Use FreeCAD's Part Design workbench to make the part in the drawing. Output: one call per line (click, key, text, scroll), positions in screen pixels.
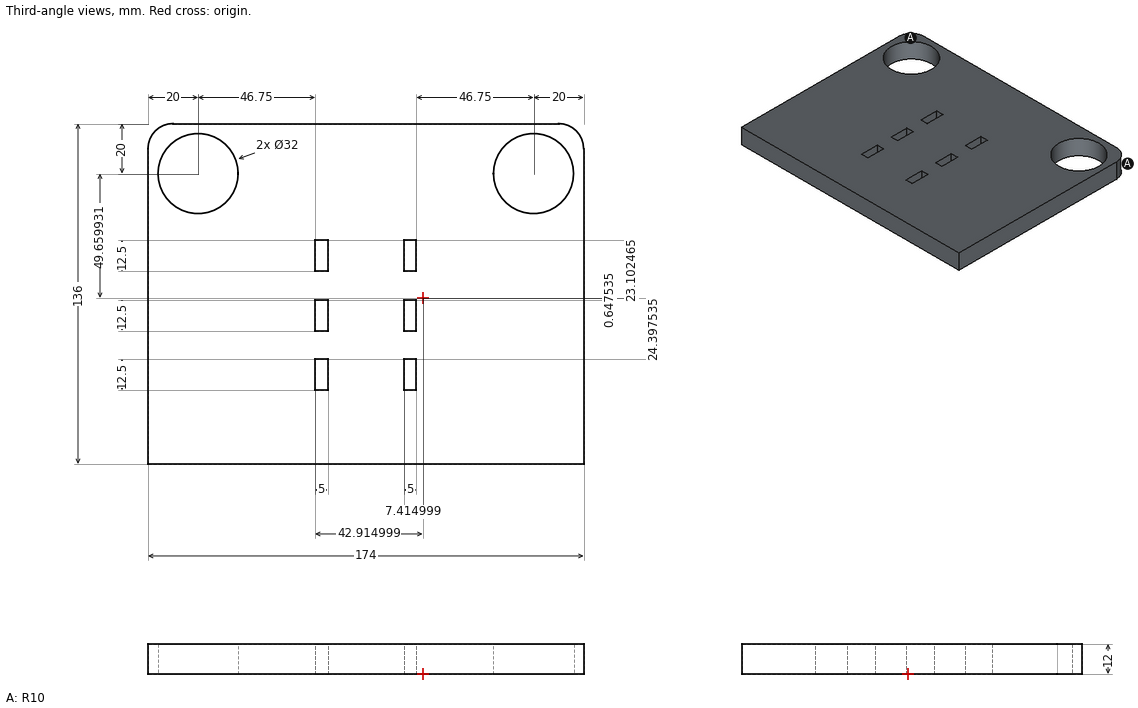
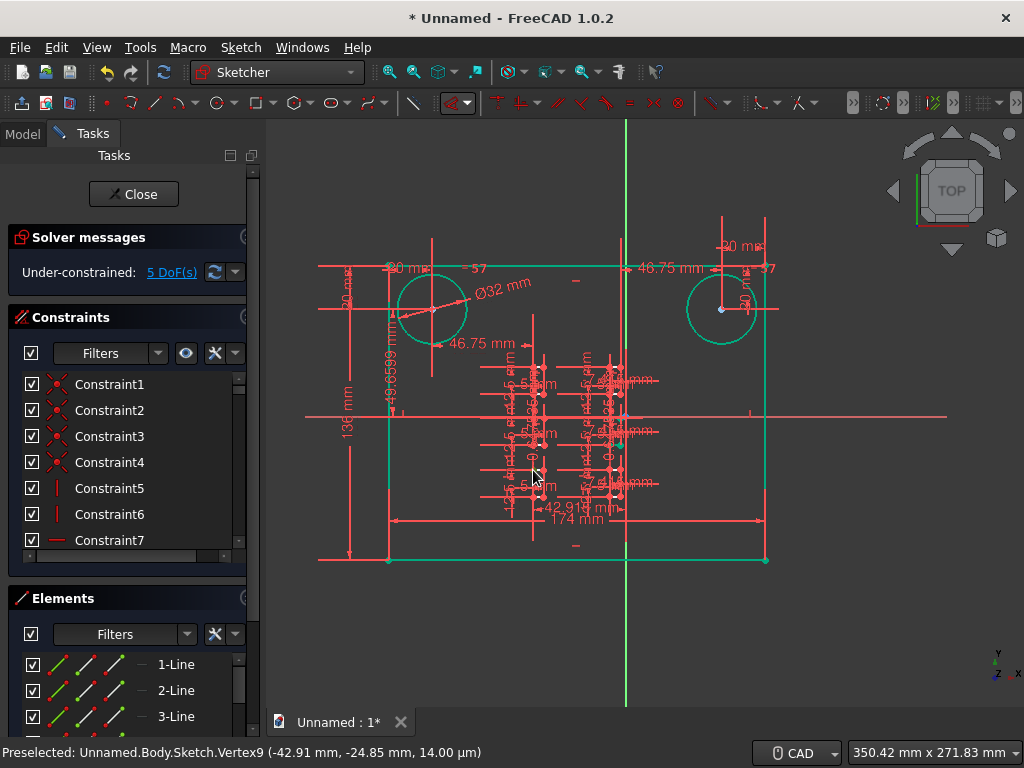
click(470, 104)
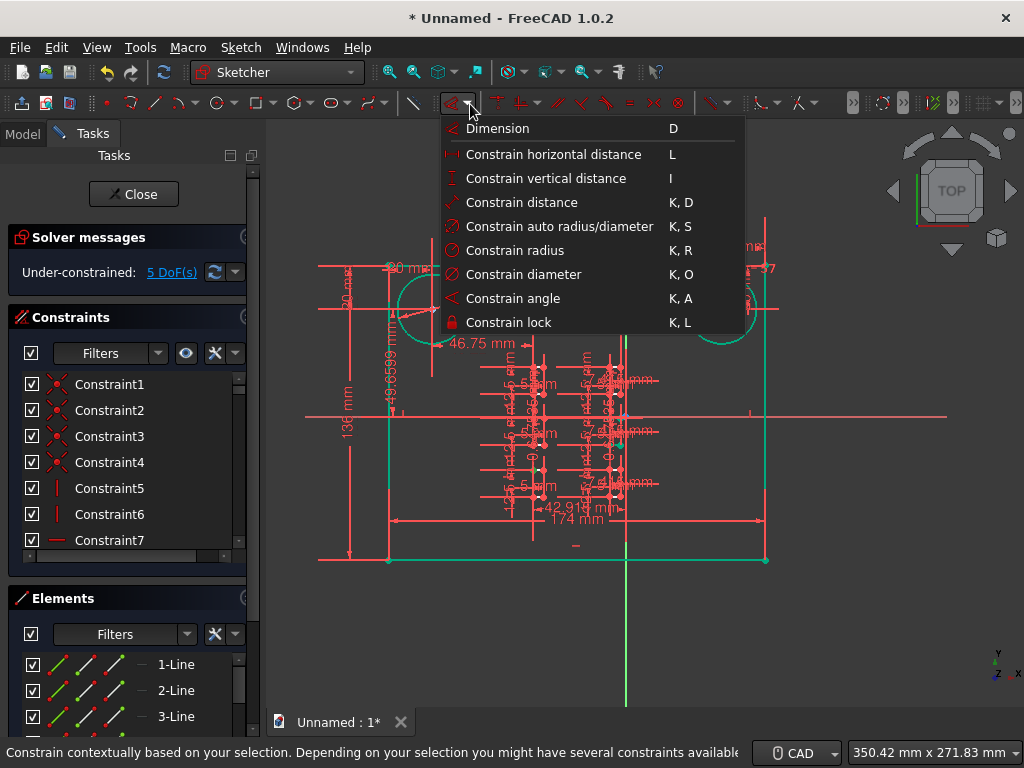
click(593, 178)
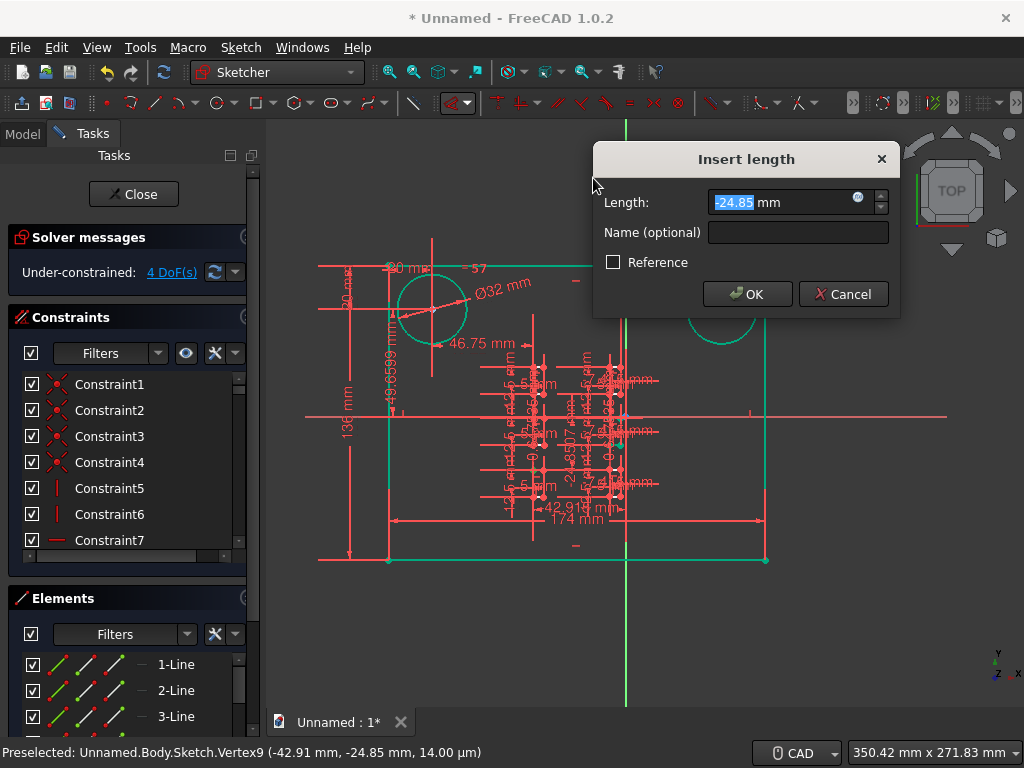
text(-24.397535)
key(Return)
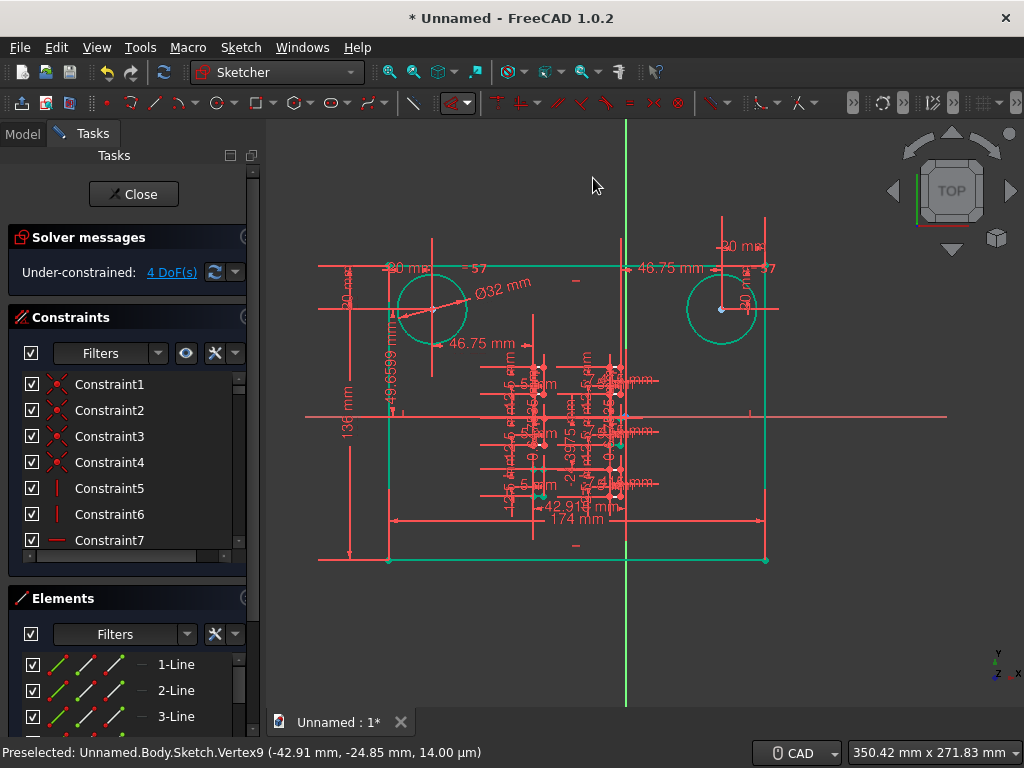
click(533, 418)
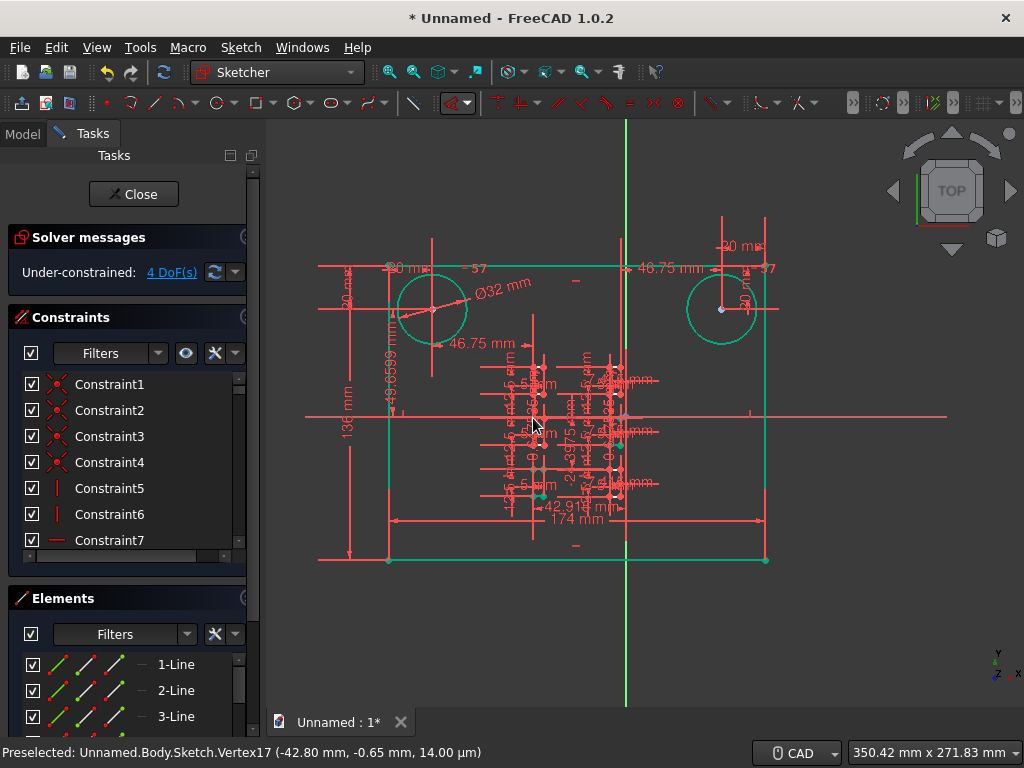
key(l)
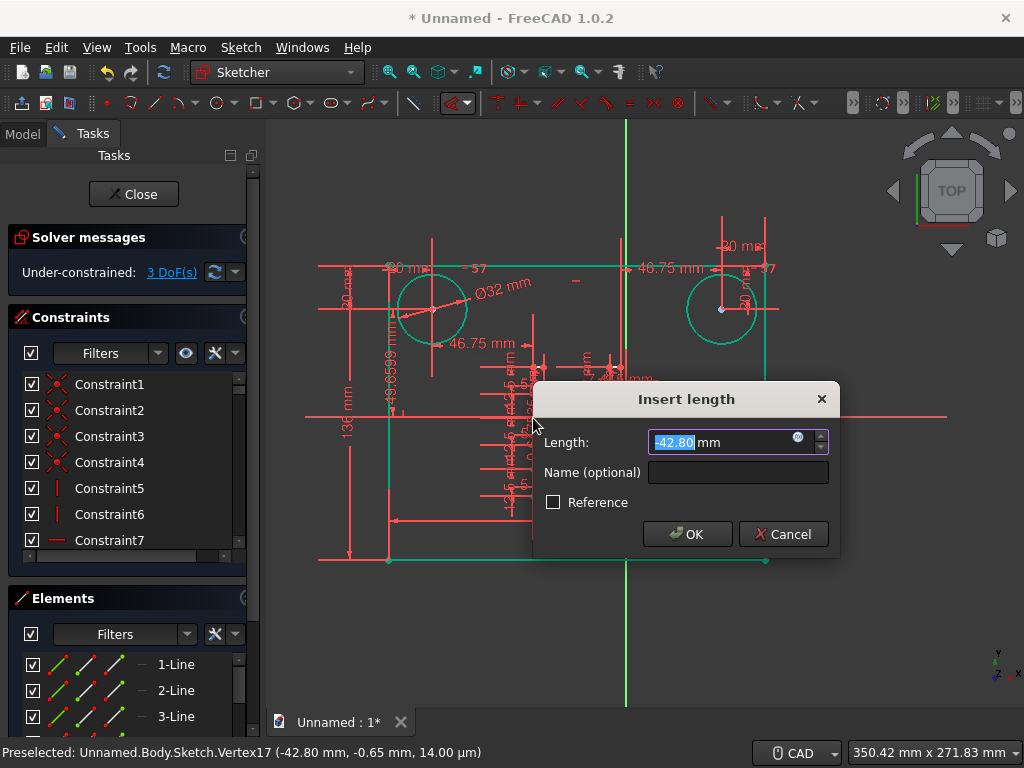
text(-42.914999)
key(Return)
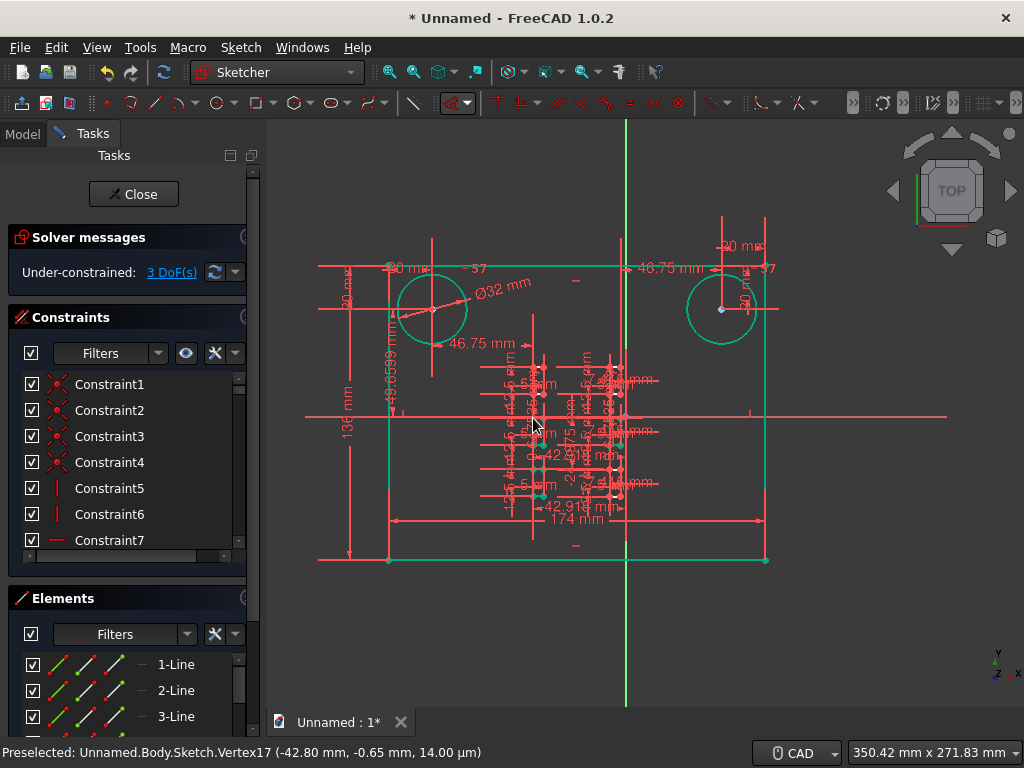
click(610, 470)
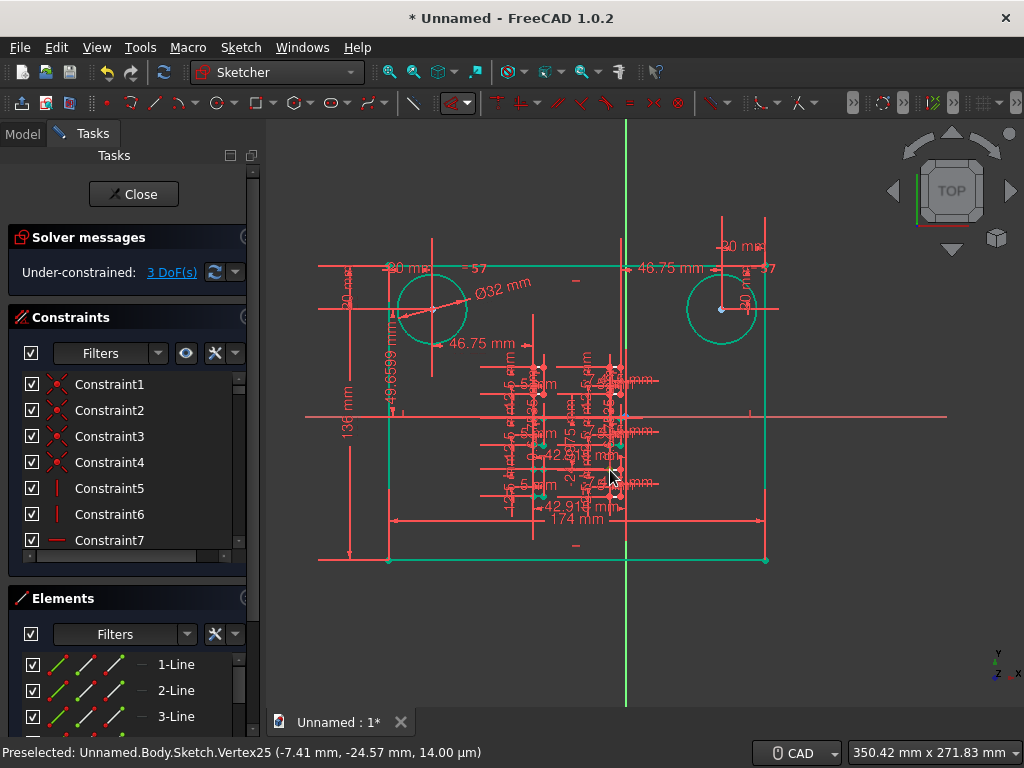
key(i)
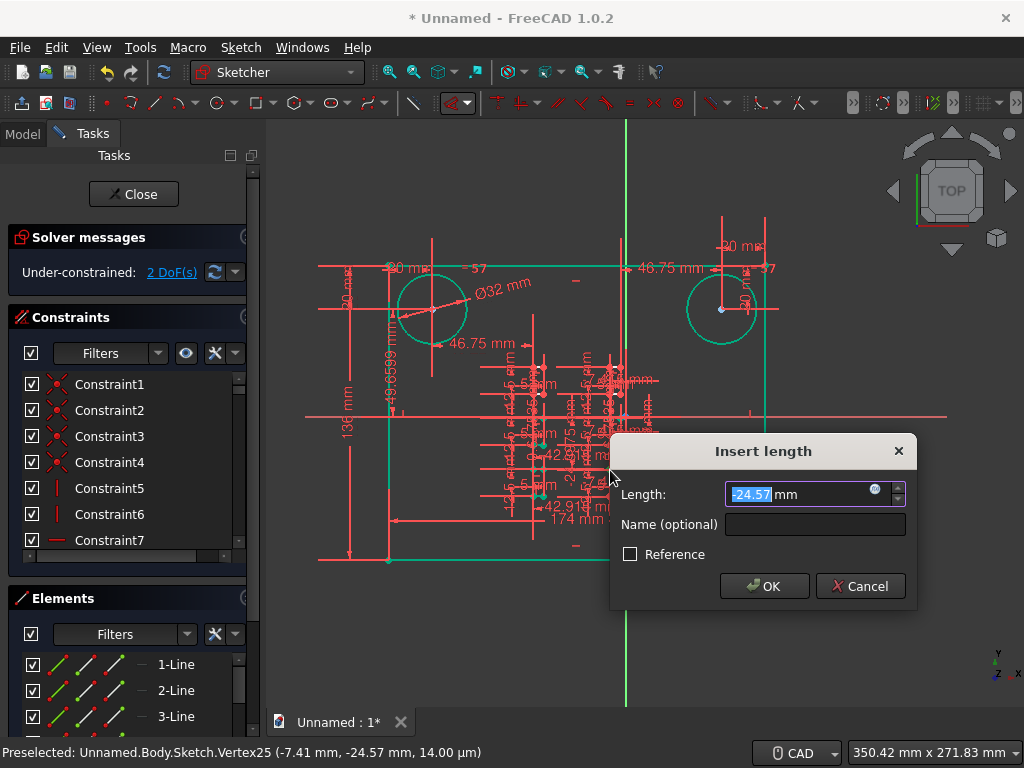
text(-24.397535)
key(Return)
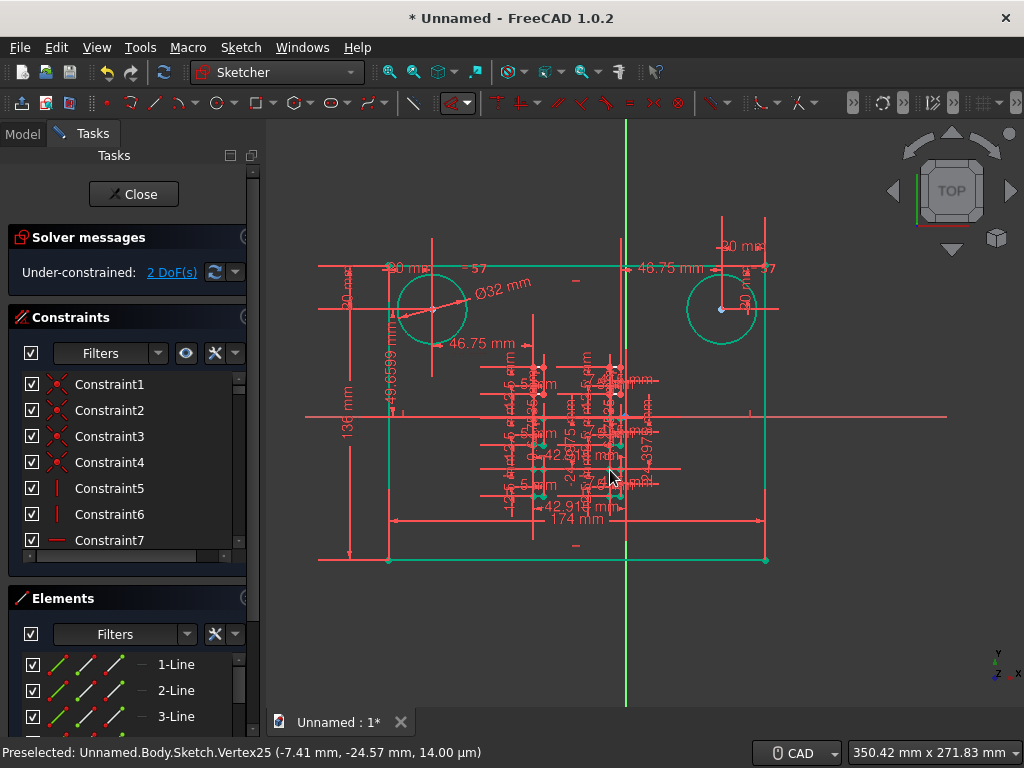
click(533, 367)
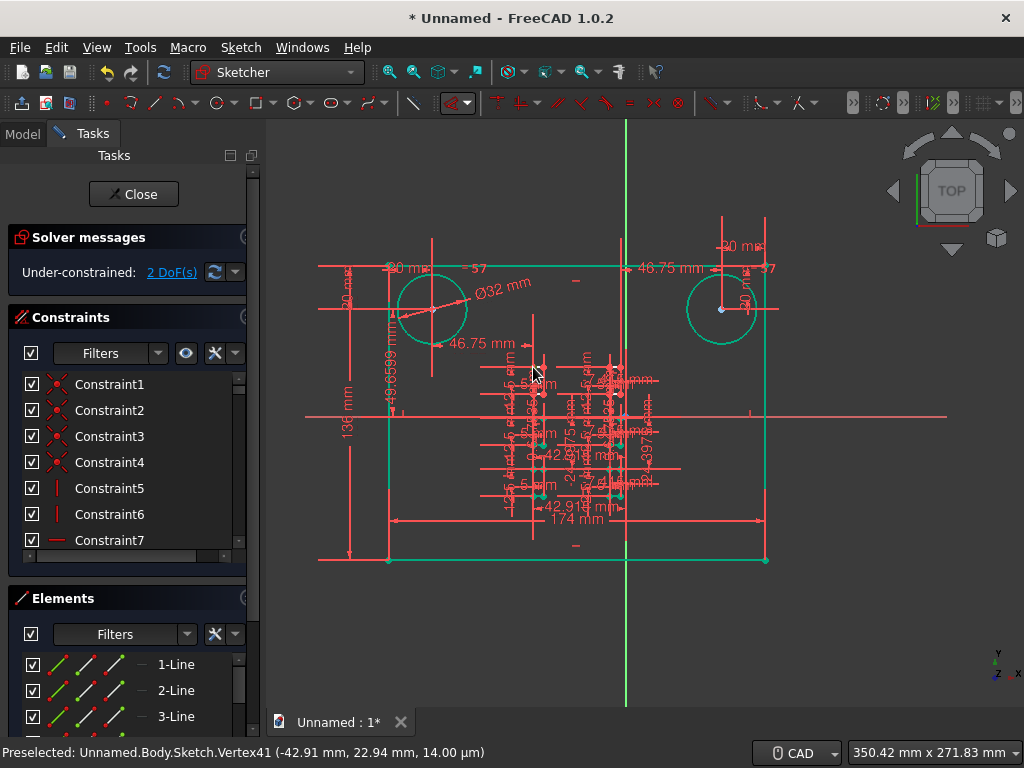
click(470, 104)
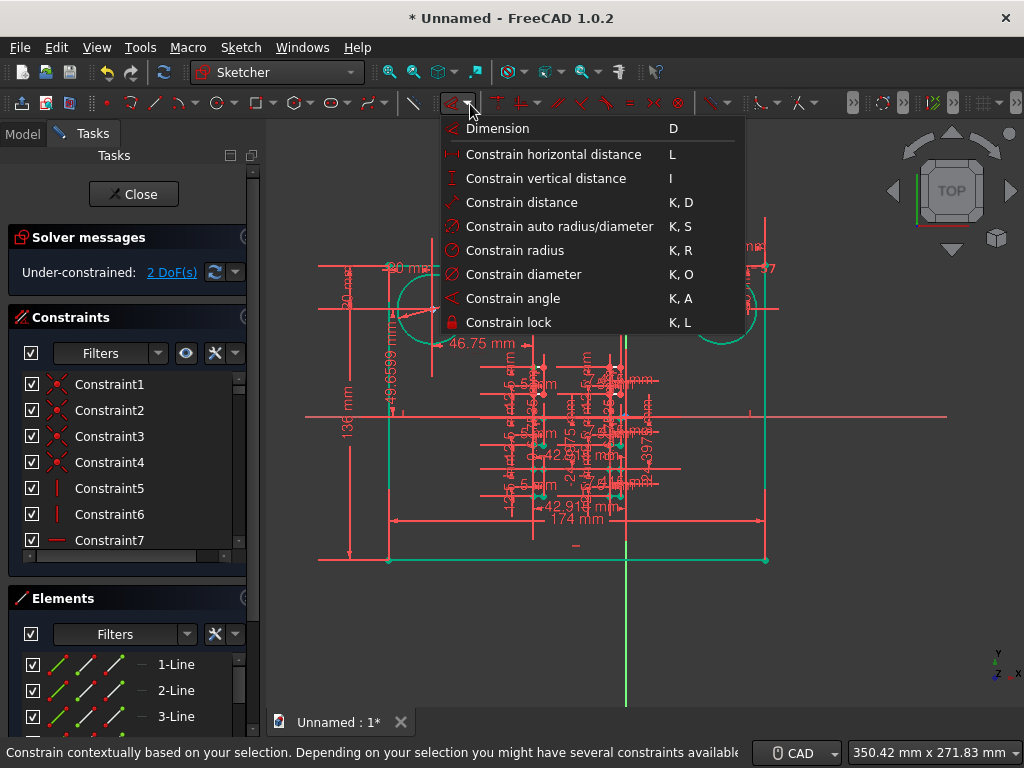
click(593, 178)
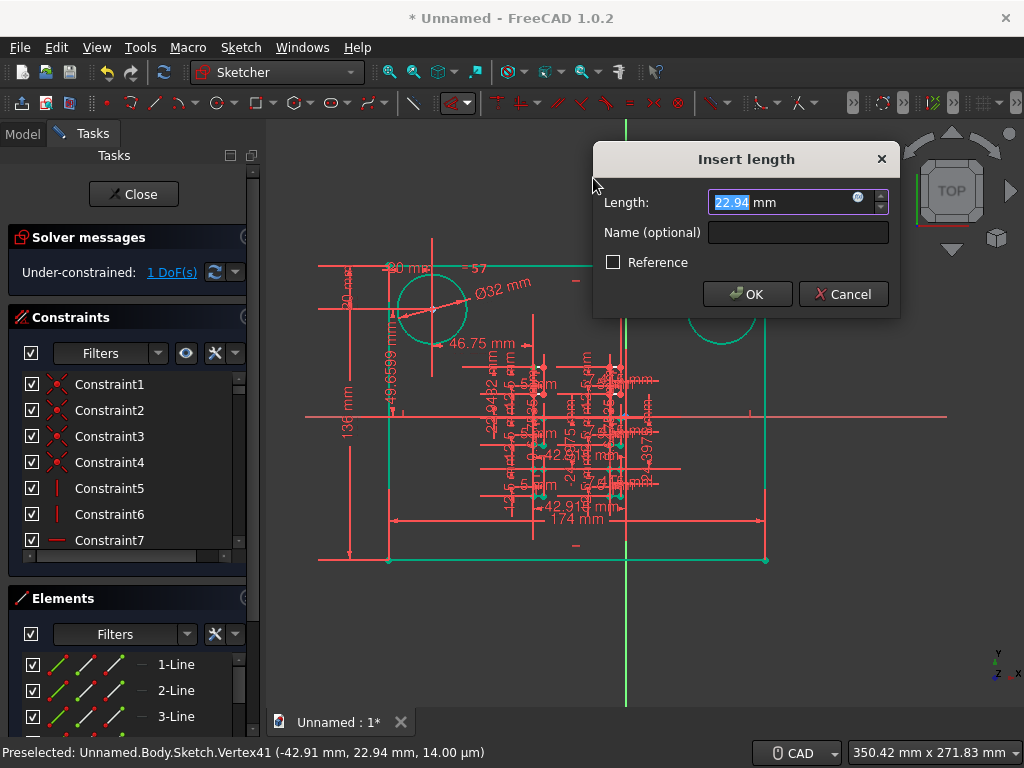
text(23.102465)
key(Return)